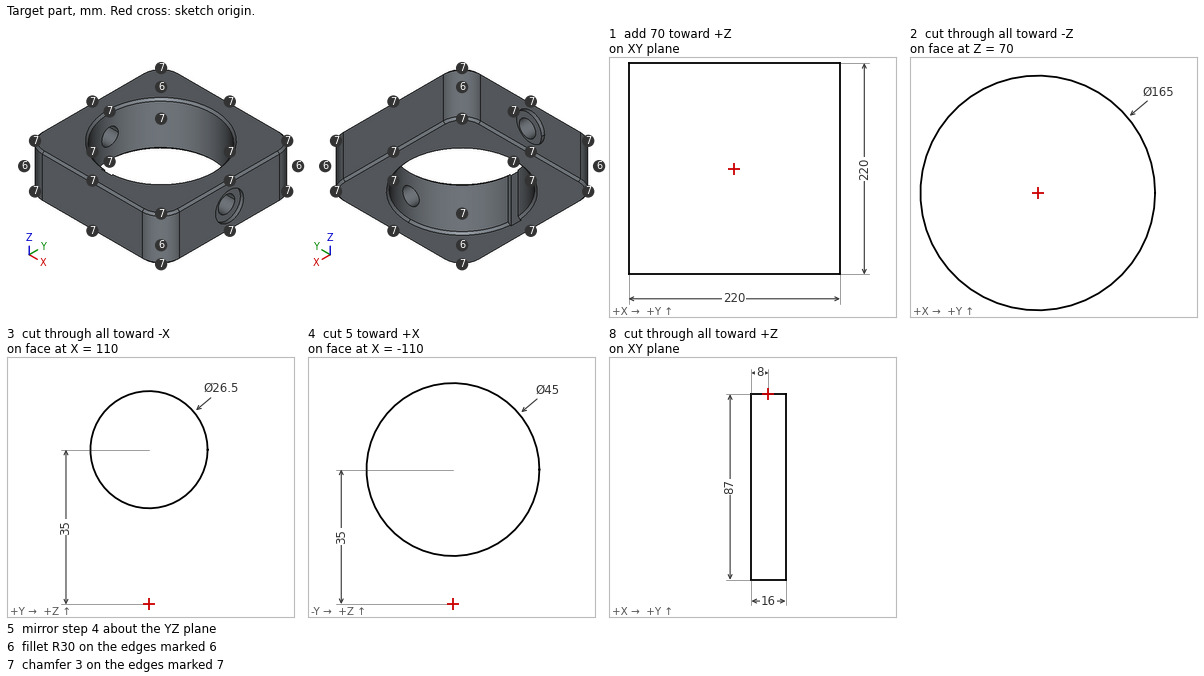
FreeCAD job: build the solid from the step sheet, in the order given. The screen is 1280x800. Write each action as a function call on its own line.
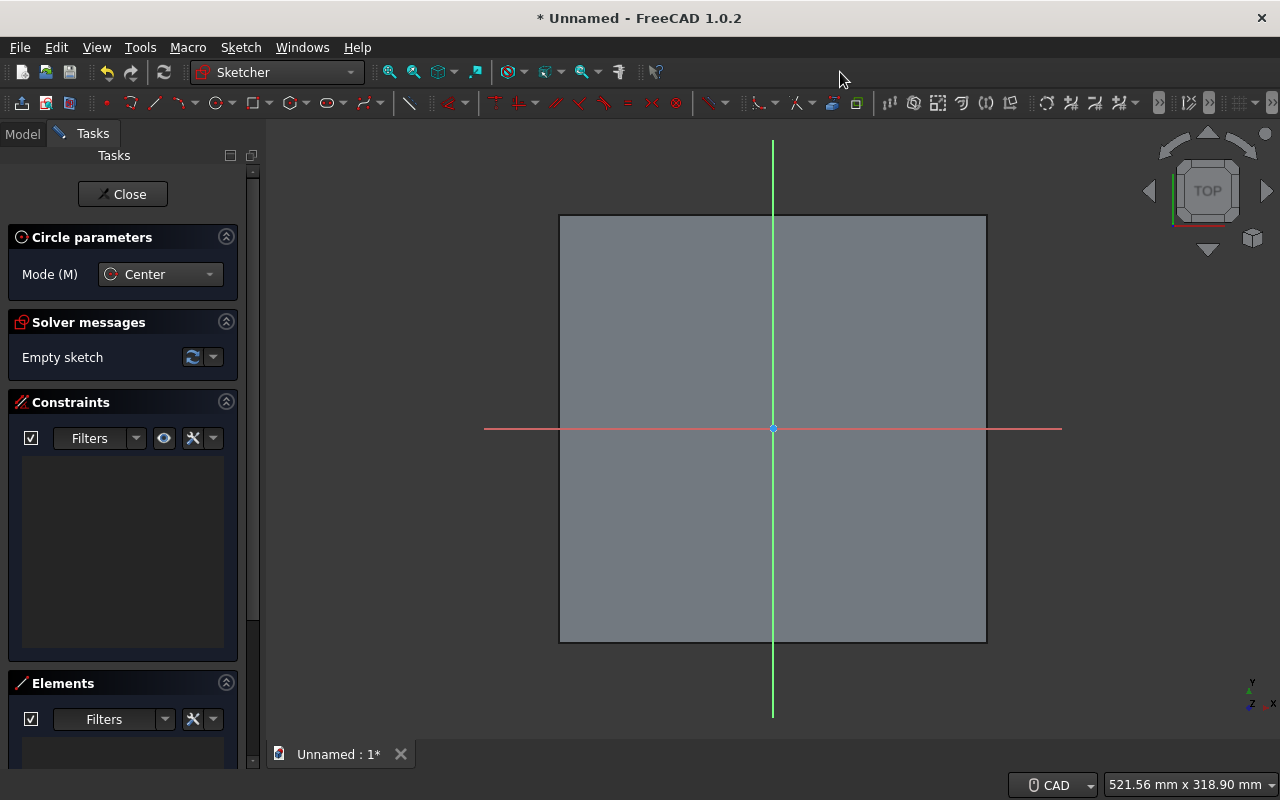
click(773, 429)
click(886, 316)
key(Escape)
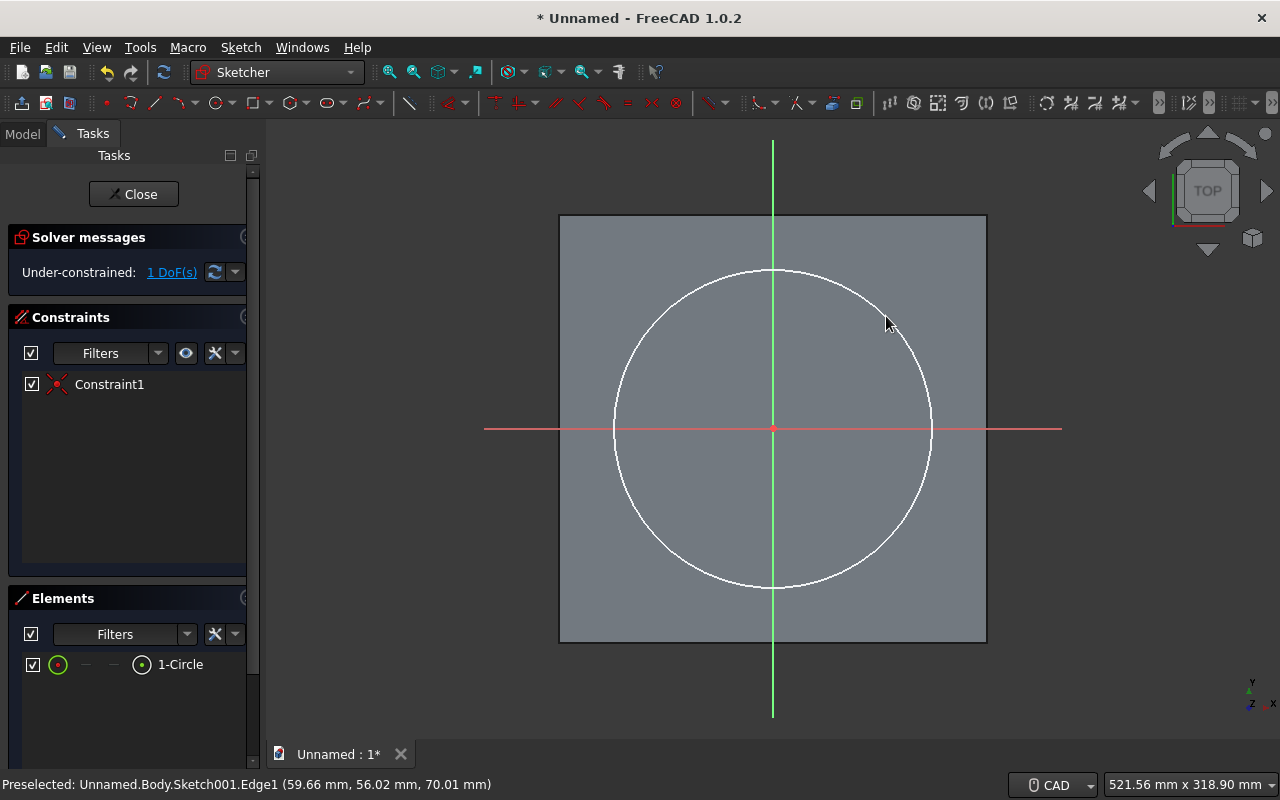
key(d)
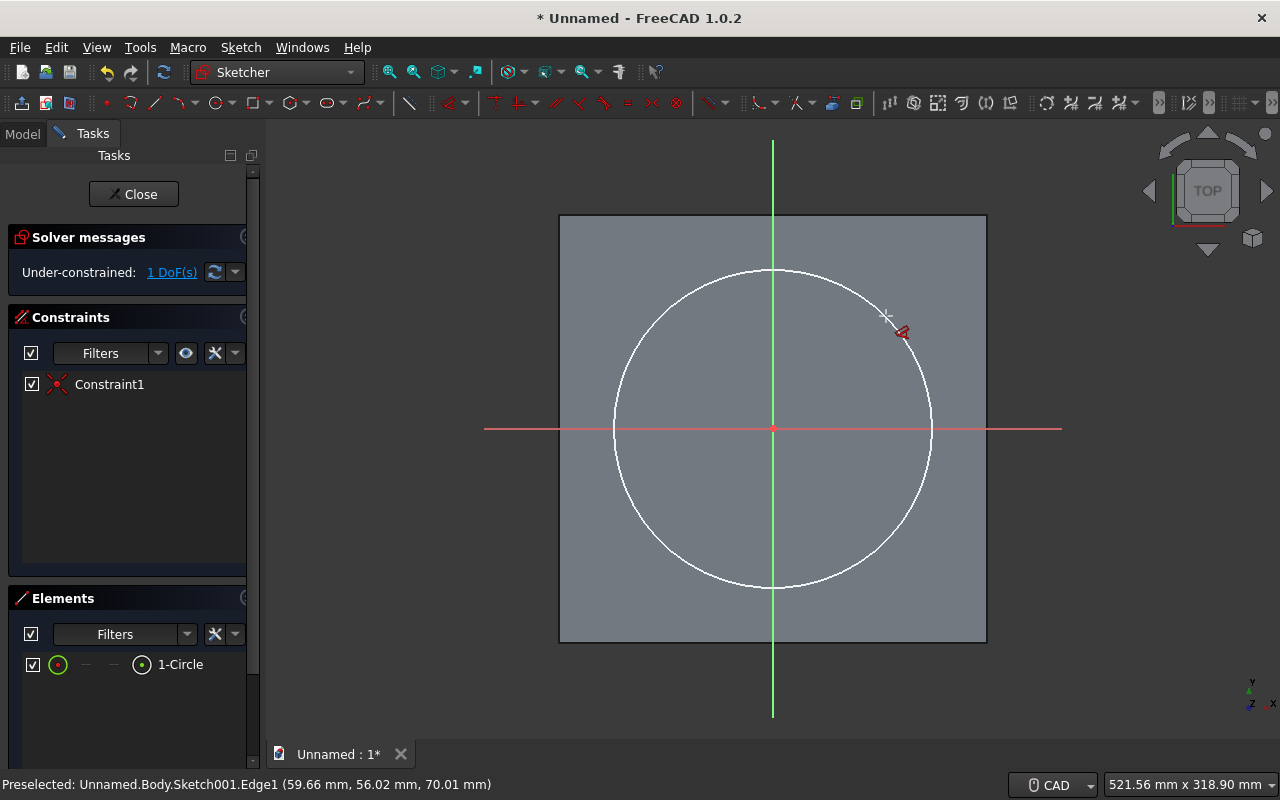
click(885, 316)
click(908, 293)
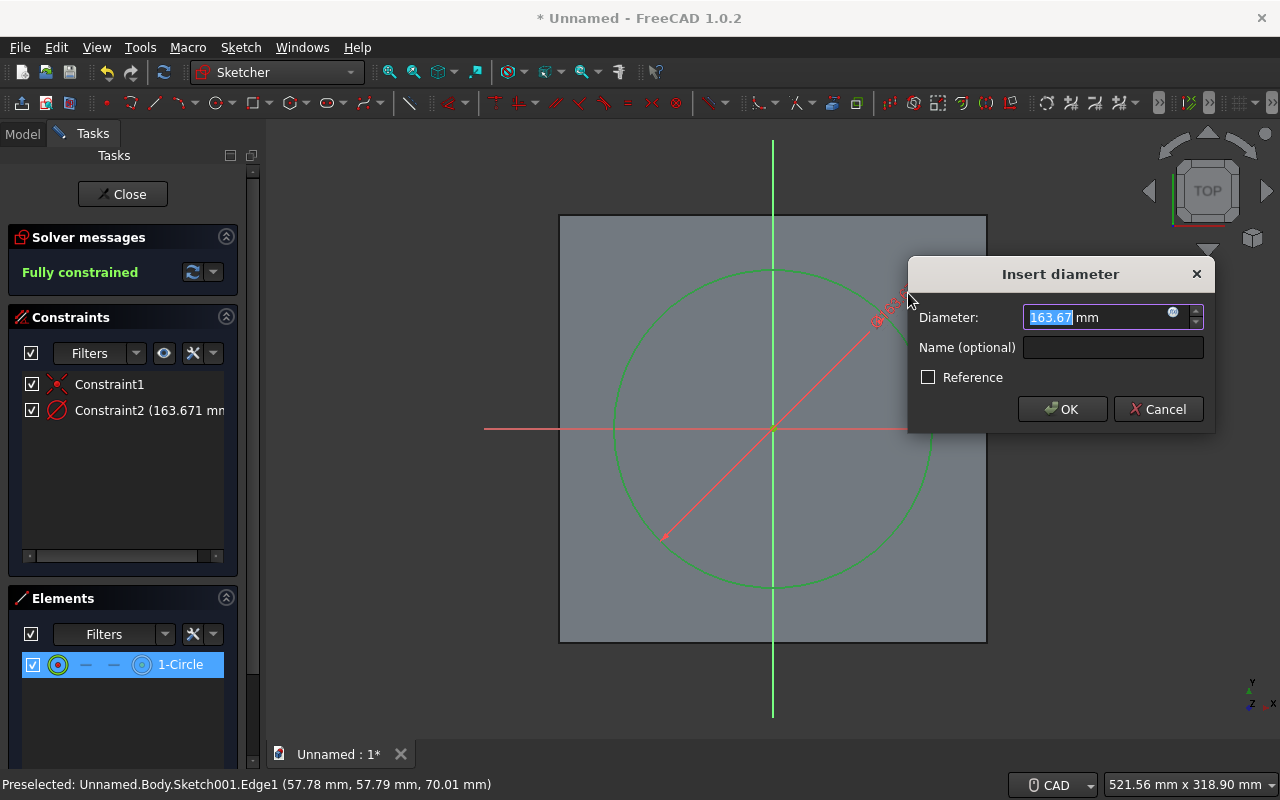
text(165)
key(Return)
key(Escape)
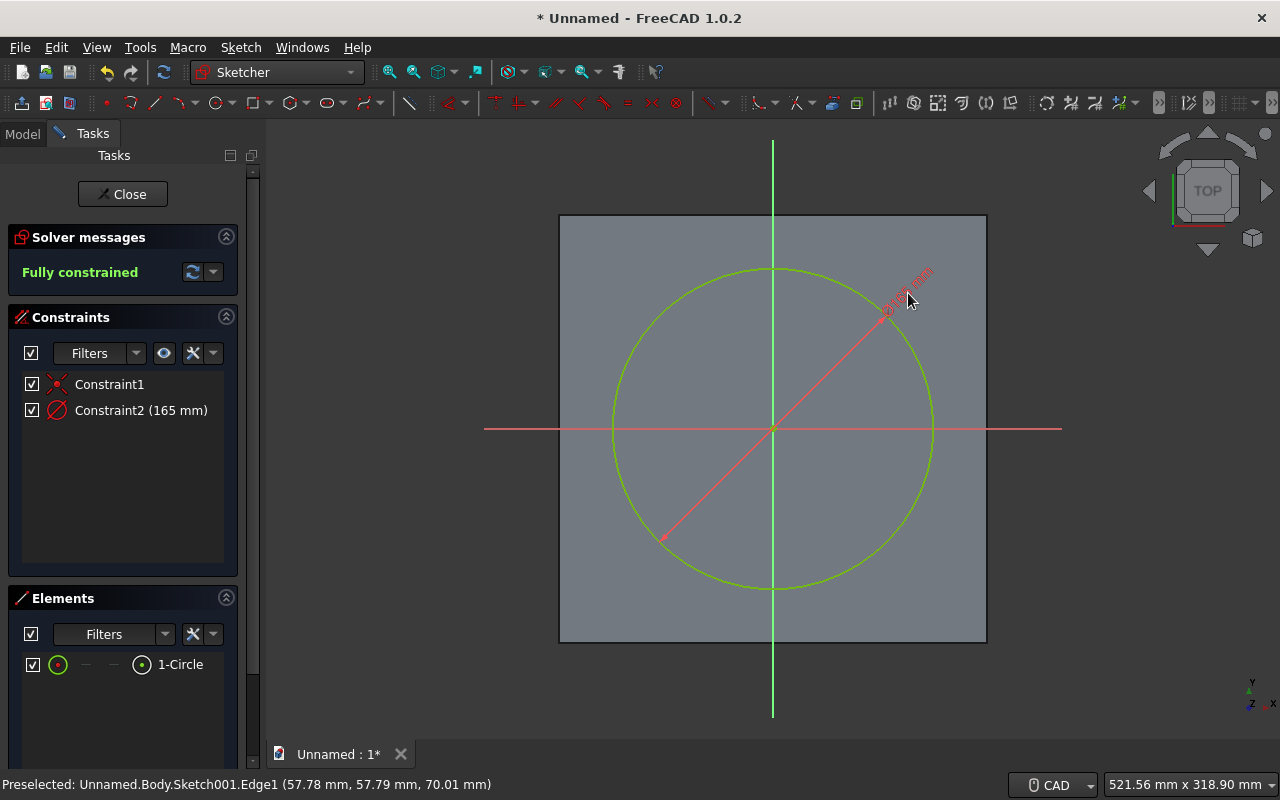
click(123, 194)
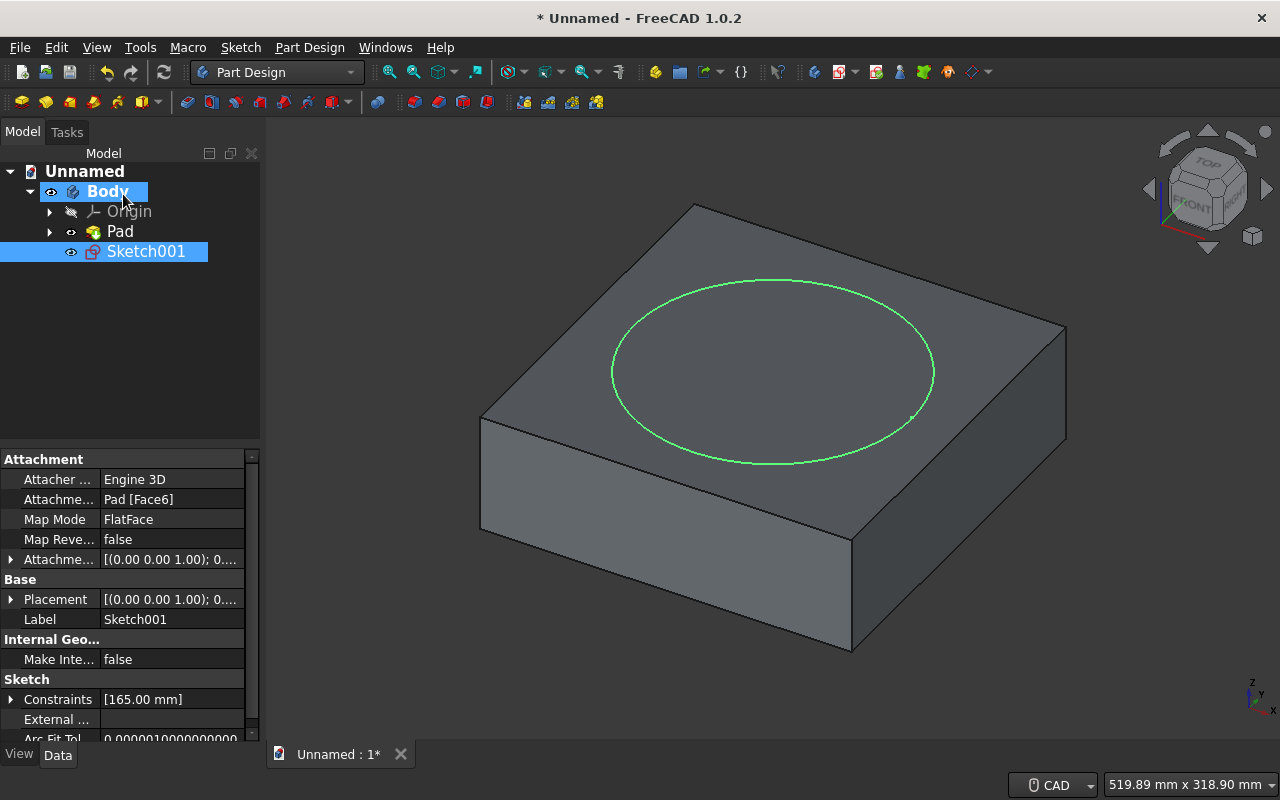
click(188, 102)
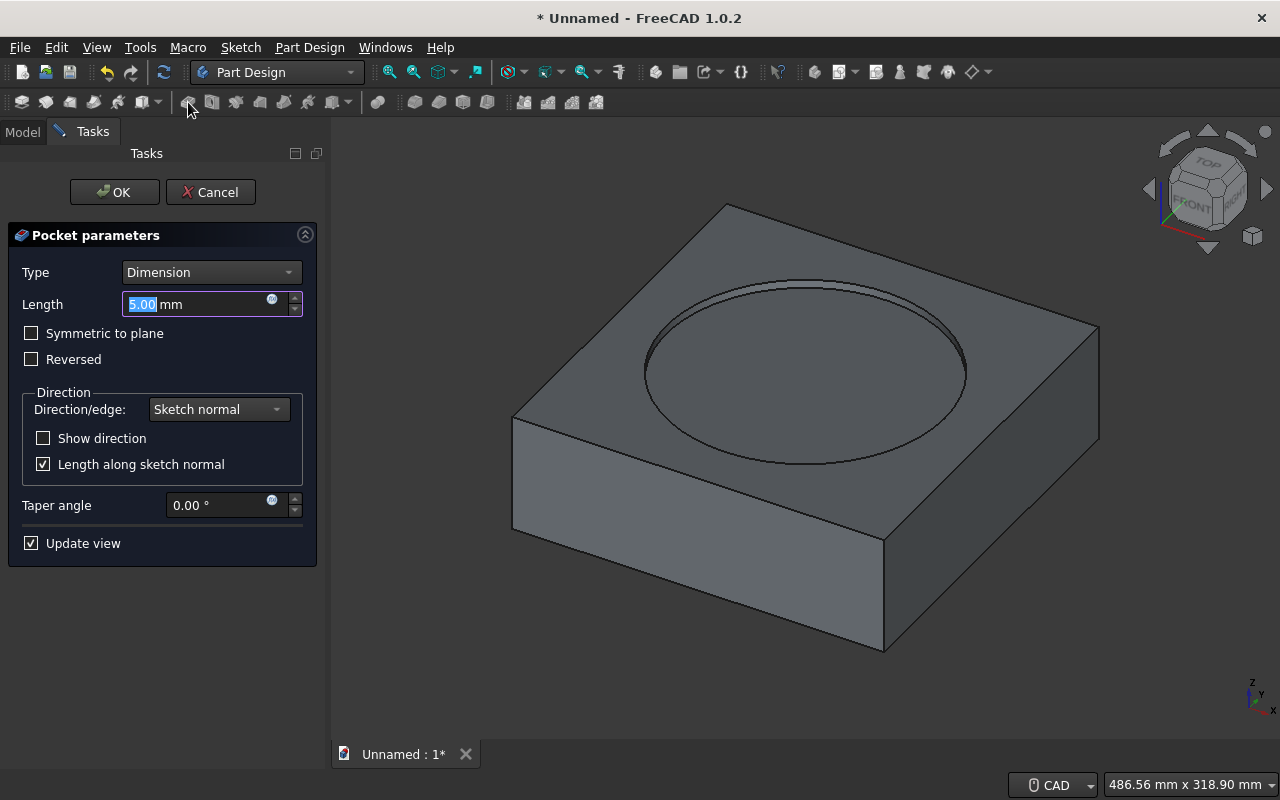
click(212, 272)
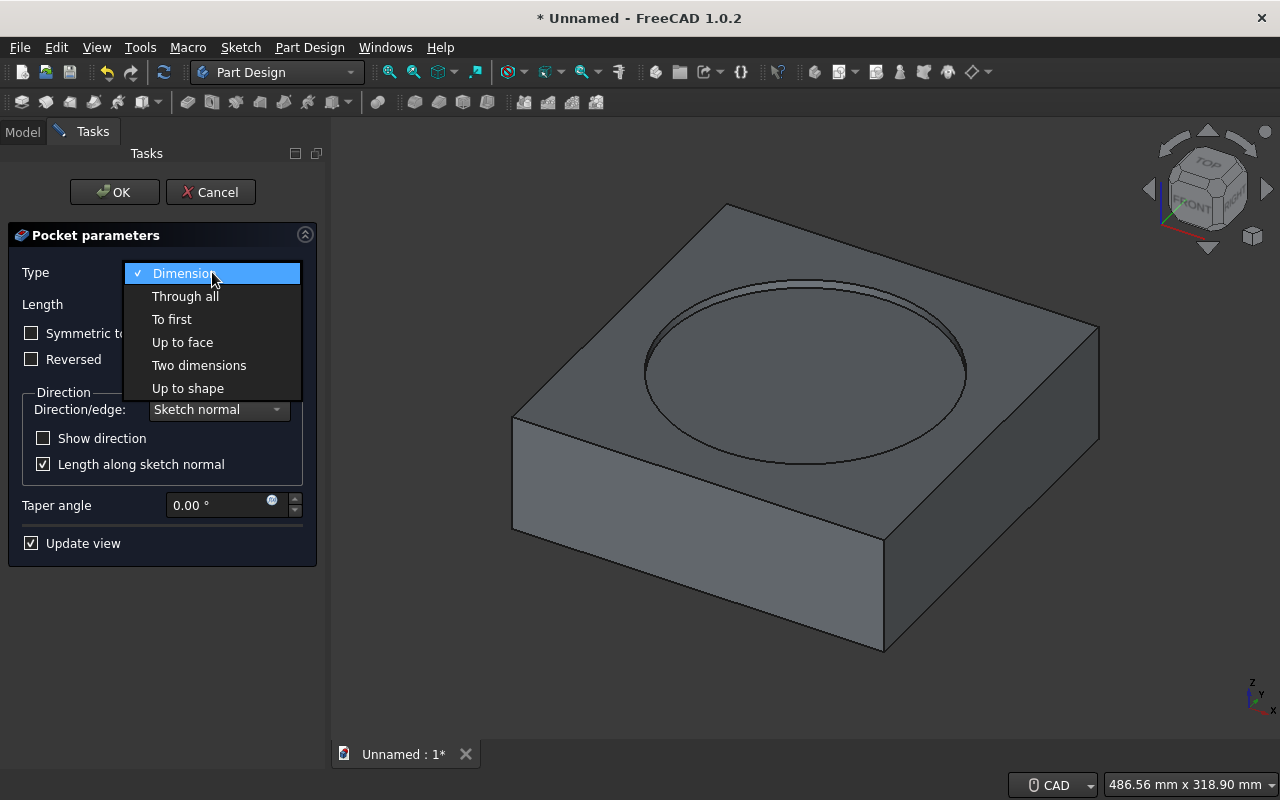
click(212, 296)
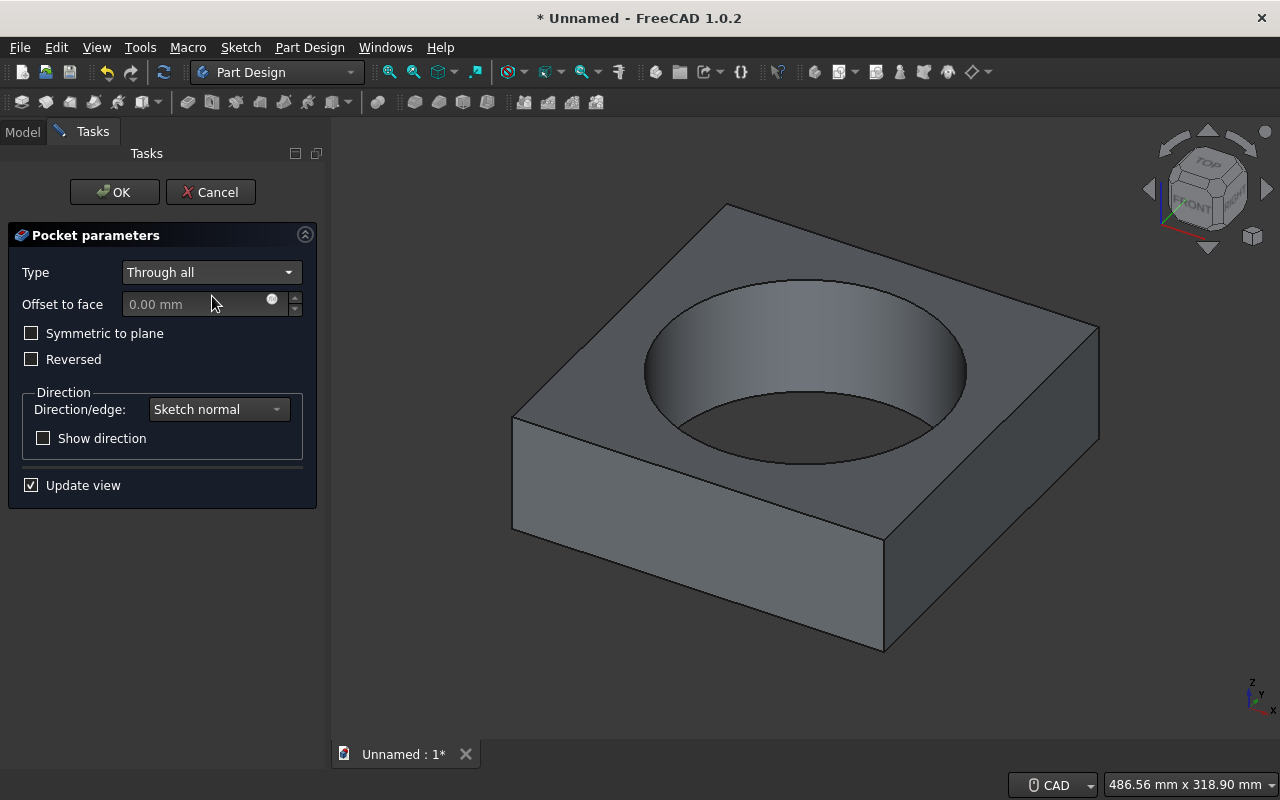
click(115, 192)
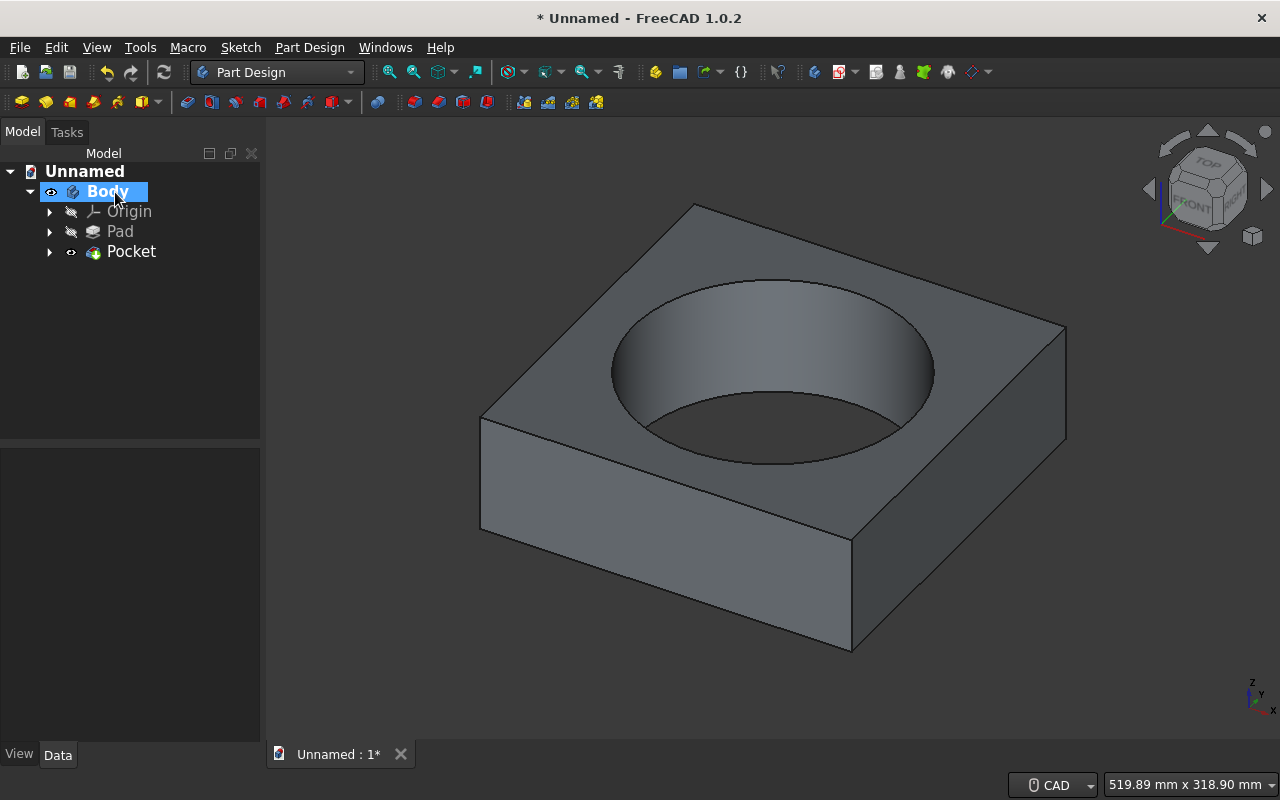
click(1020, 428)